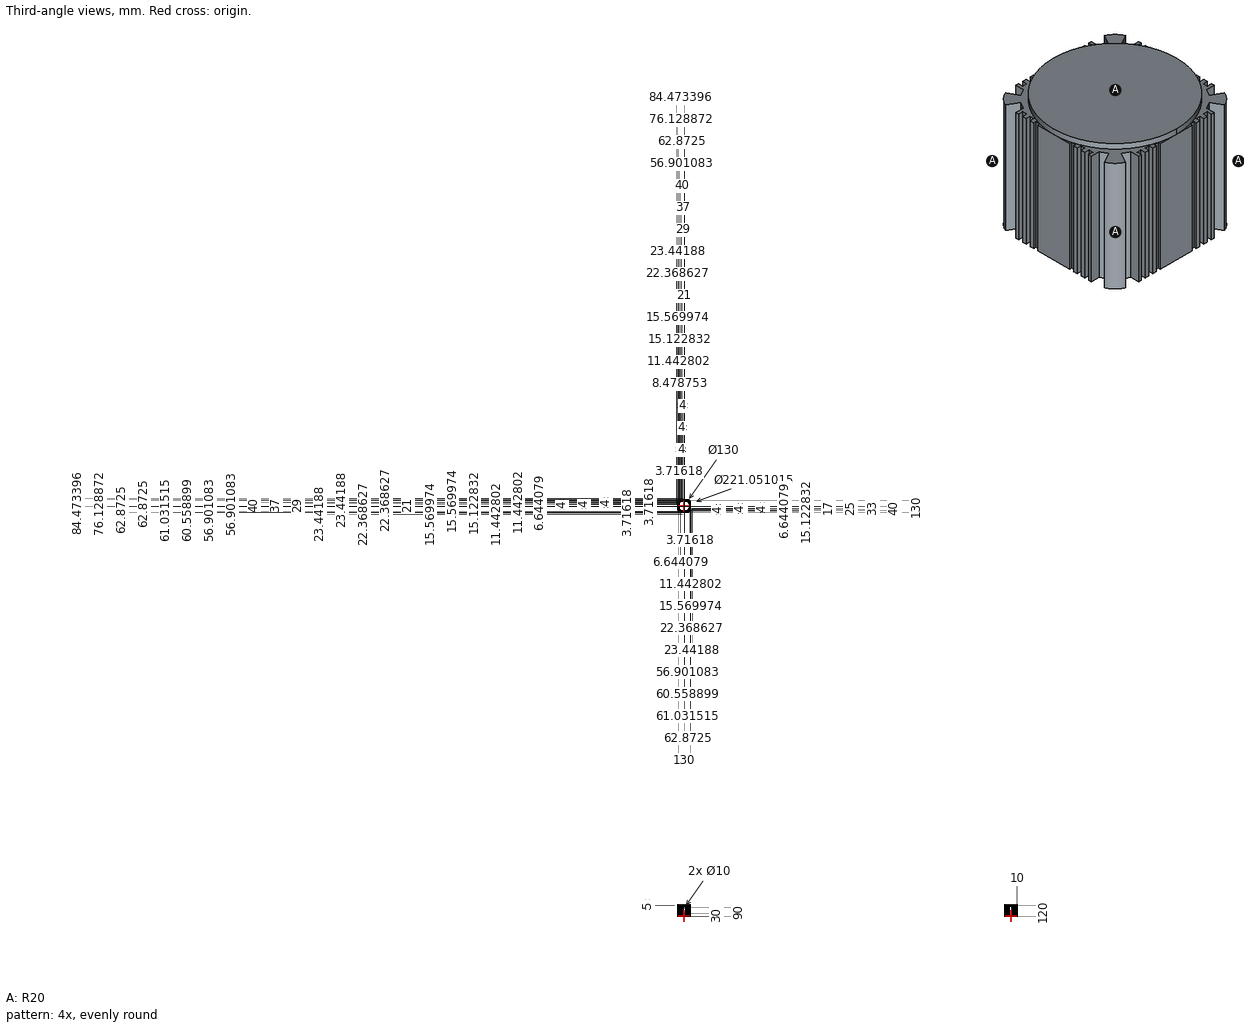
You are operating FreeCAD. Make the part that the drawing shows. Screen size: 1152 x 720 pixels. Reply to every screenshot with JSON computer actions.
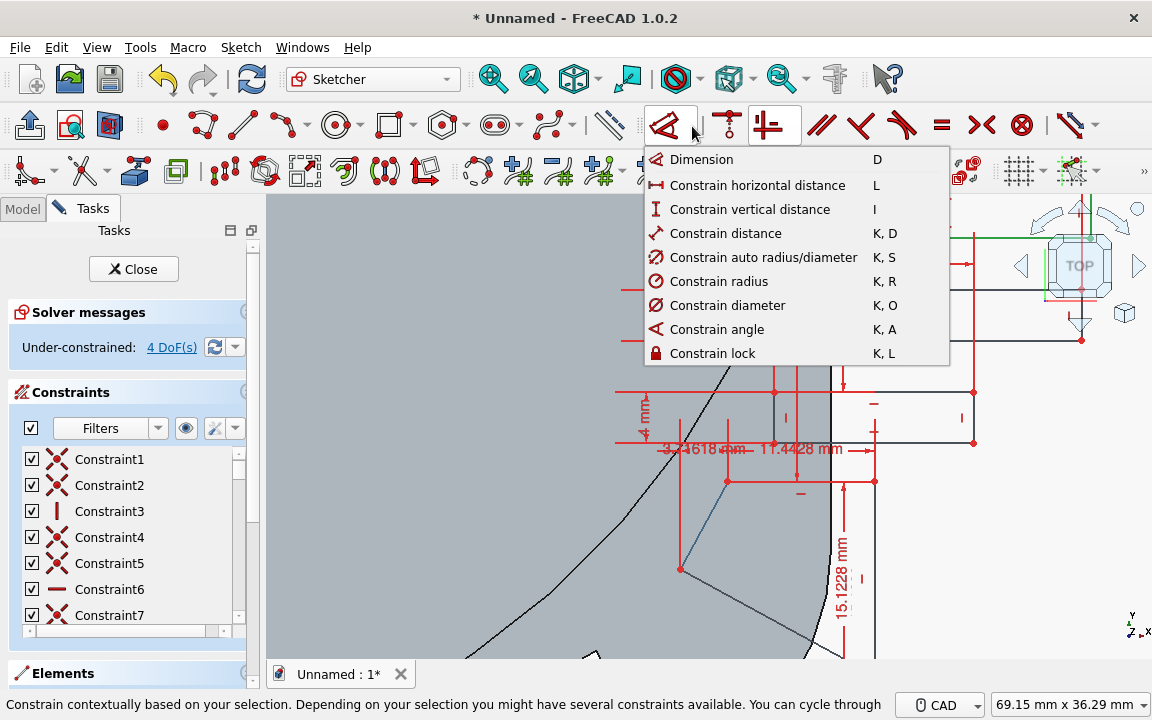
{"action": "left_click", "coordinate": [797, 209]}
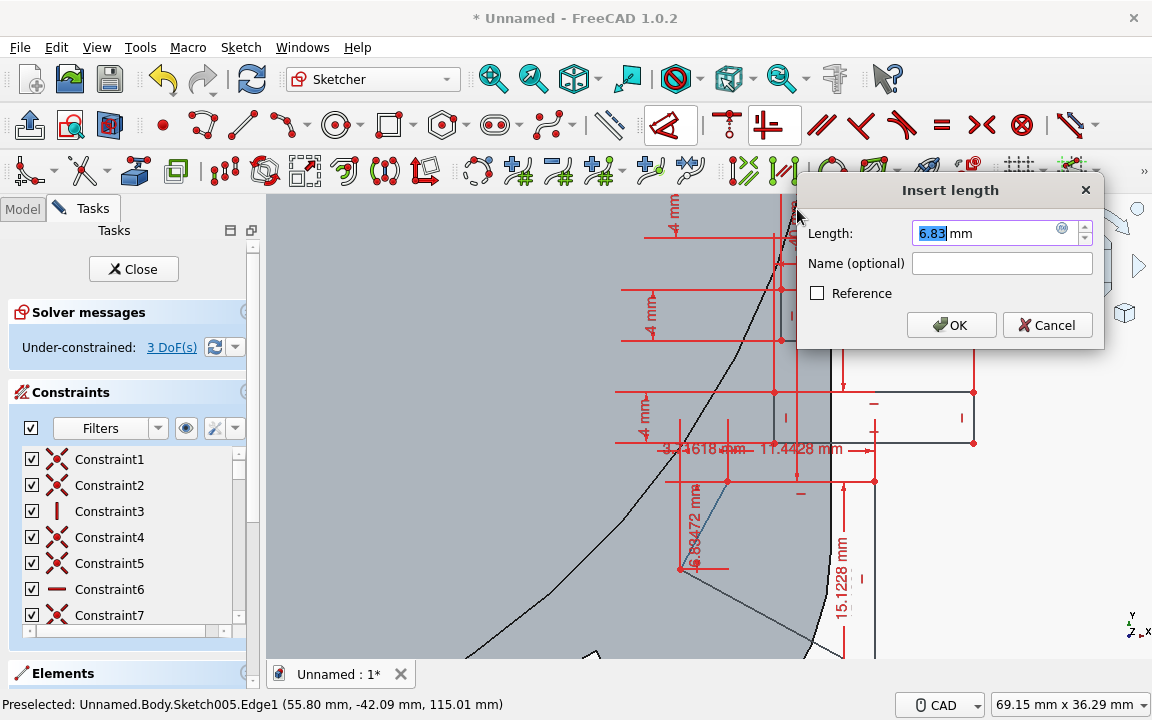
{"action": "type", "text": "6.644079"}
{"action": "key", "text": "Return"}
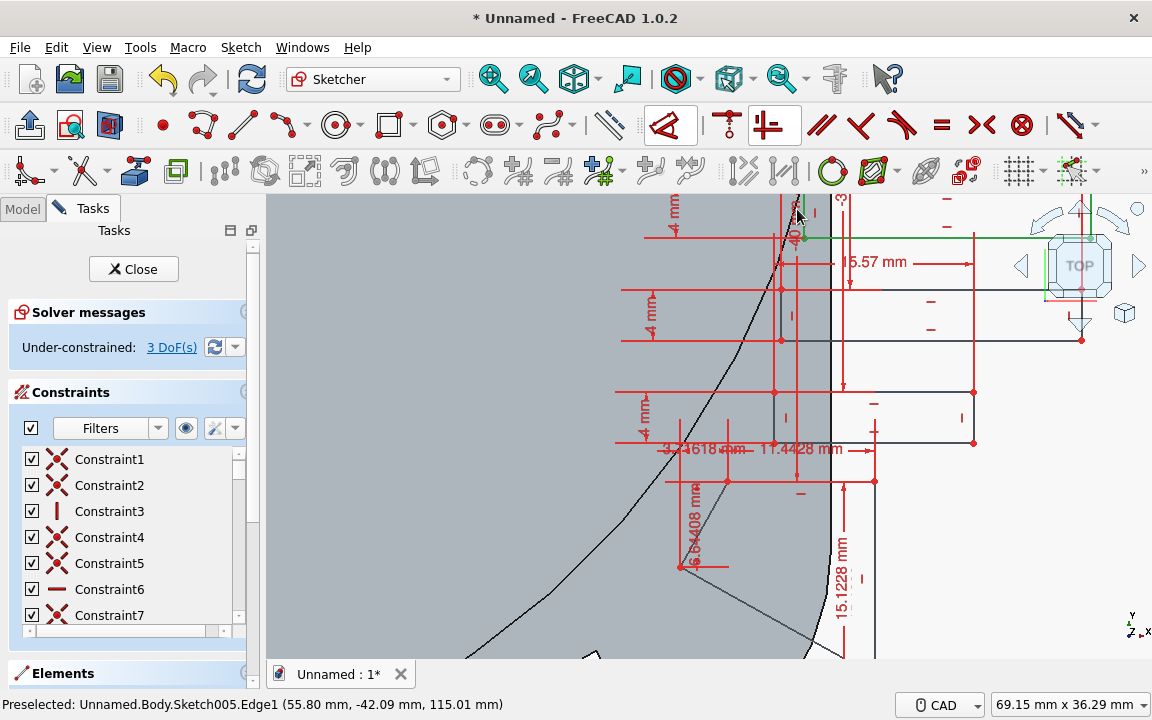
{"action": "left_click", "coordinate": [728, 482]}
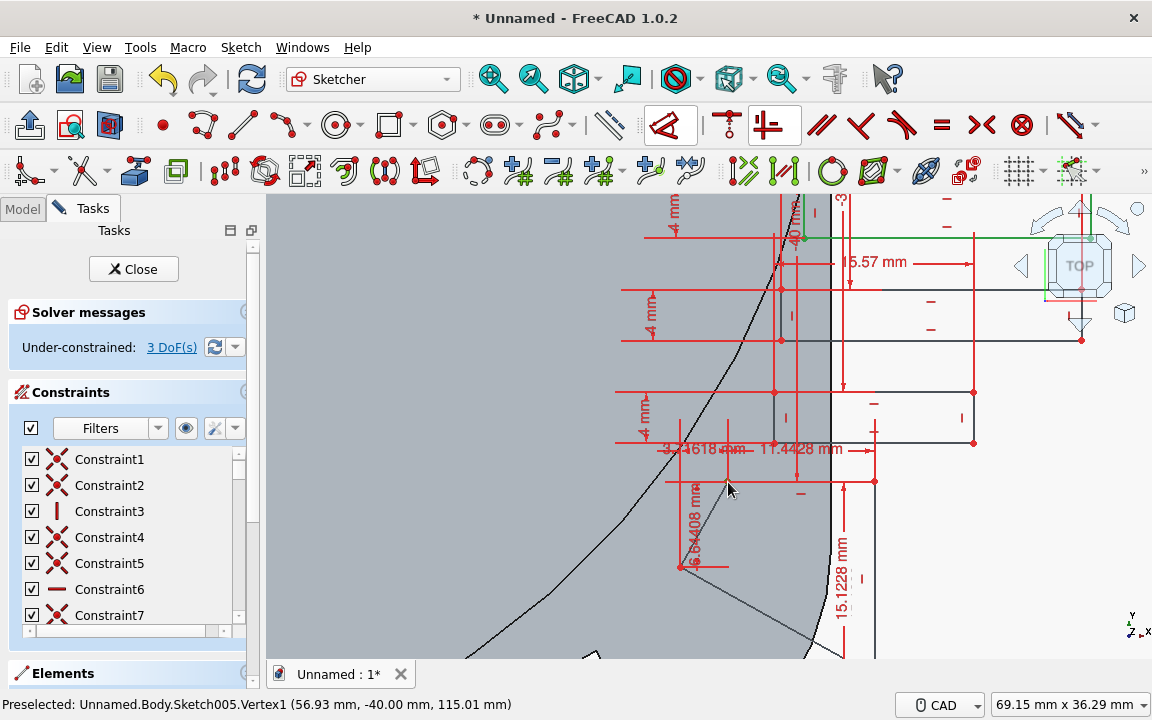
{"action": "left_click", "coordinate": [692, 126]}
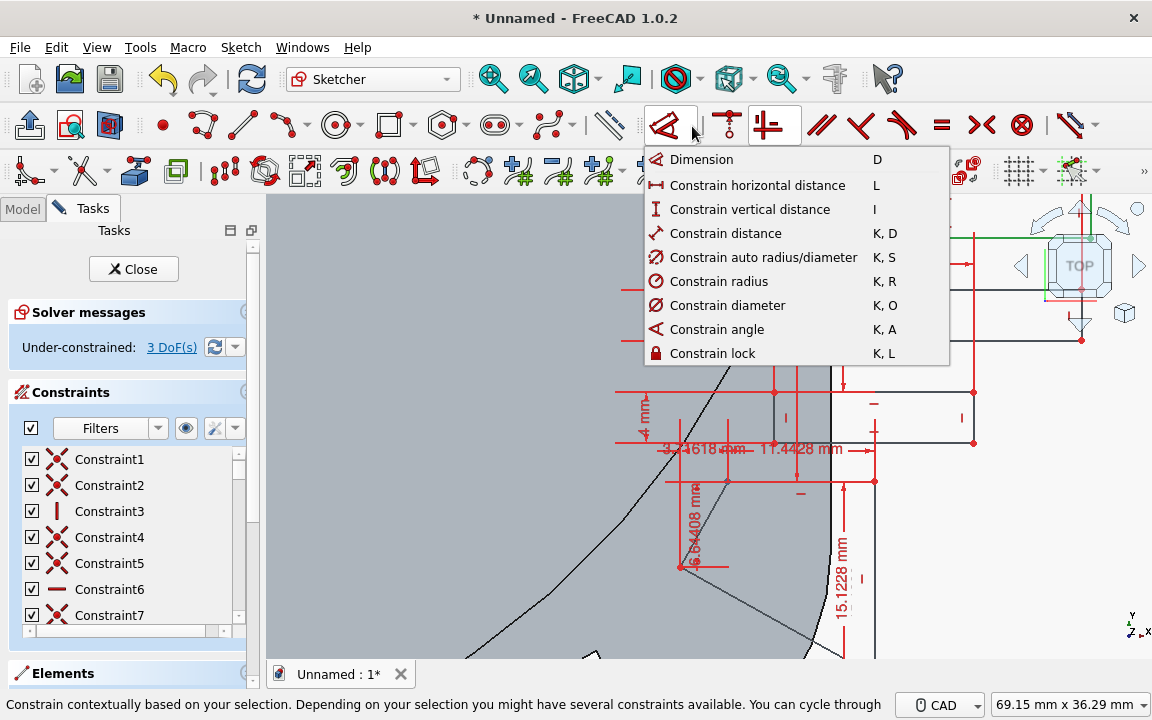
{"action": "left_click", "coordinate": [797, 185]}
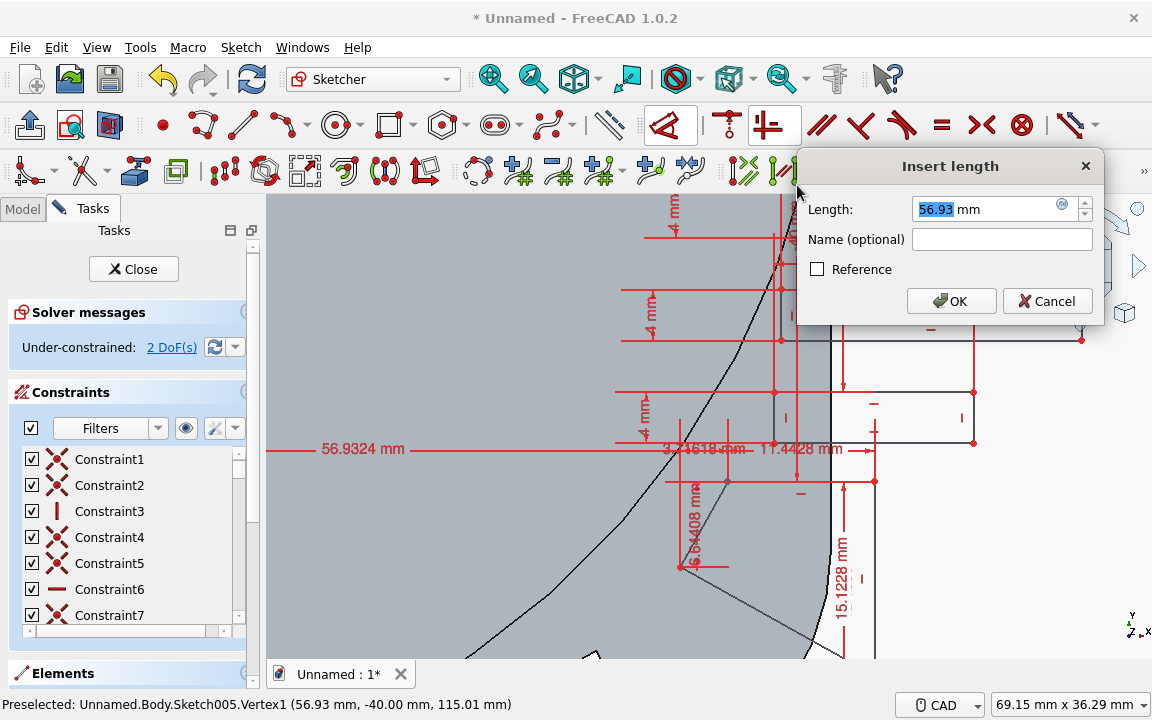
{"action": "type", "text": "56.901083"}
{"action": "key", "text": "Return"}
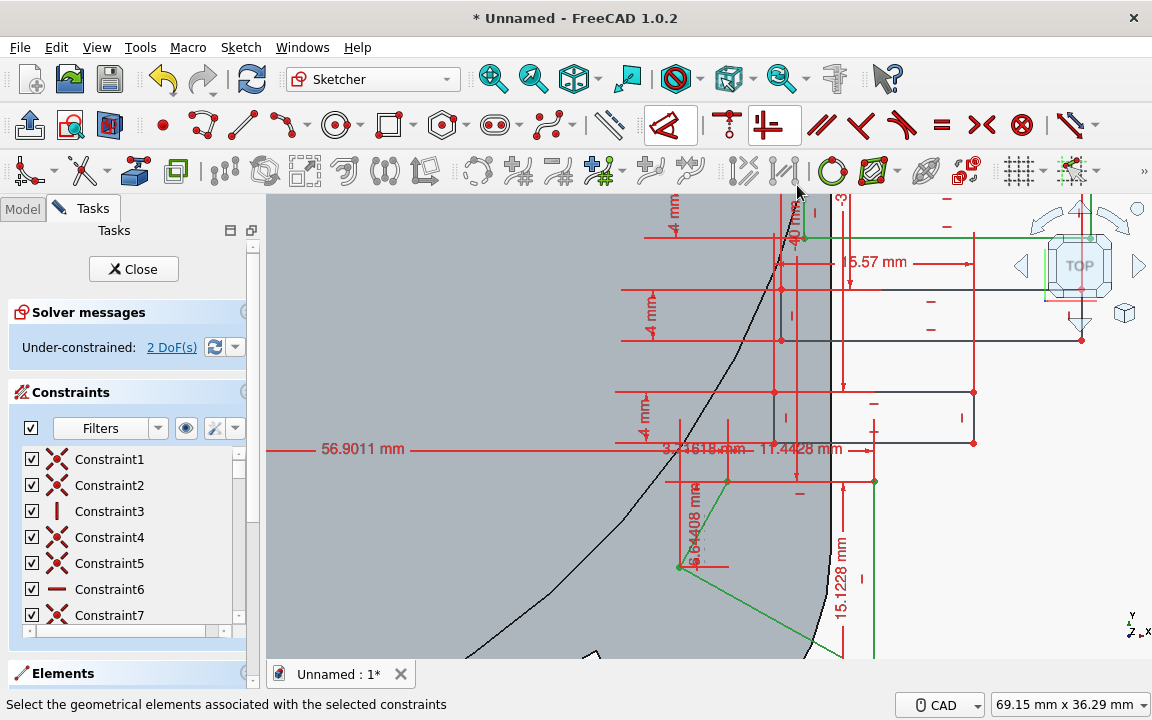
{"action": "left_click", "coordinate": [774, 392]}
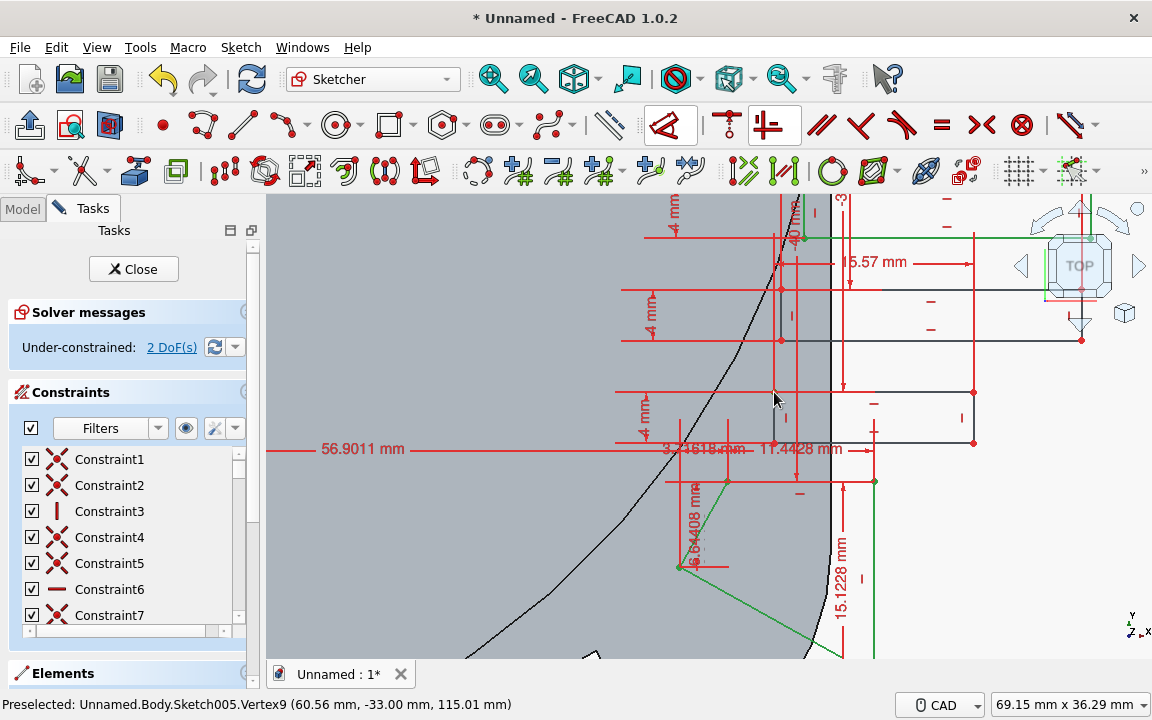
{"action": "key", "text": "l"}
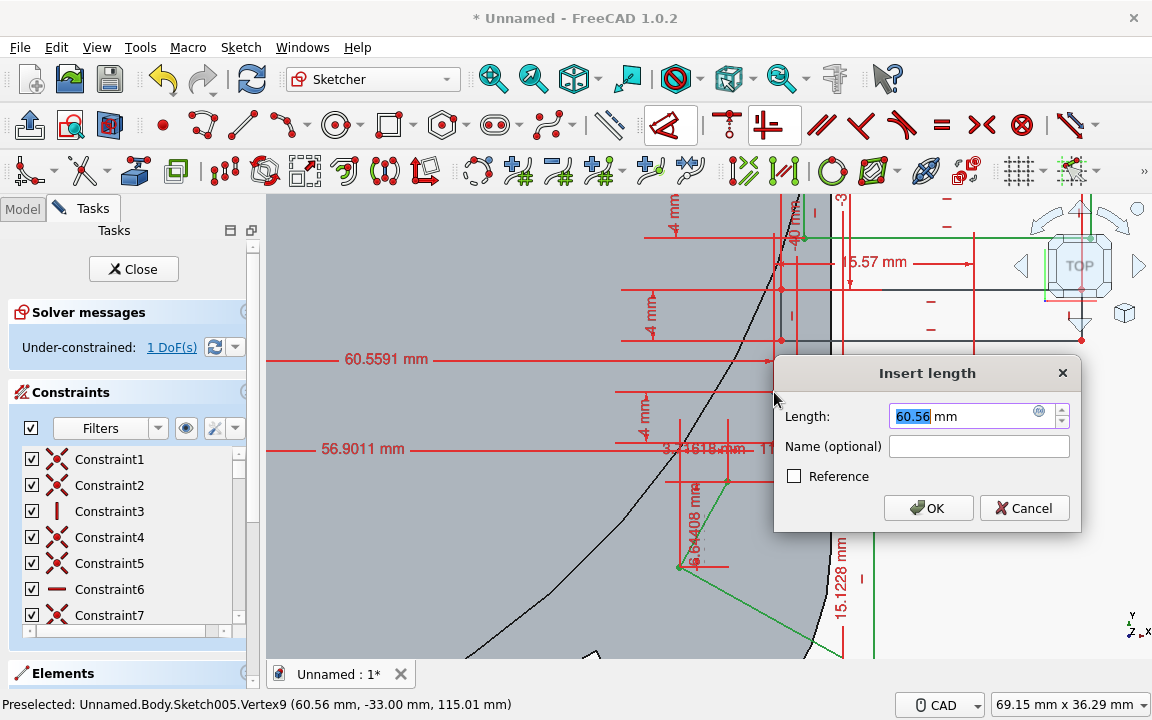
{"action": "type", "text": "60.558899"}
{"action": "key", "text": "Return"}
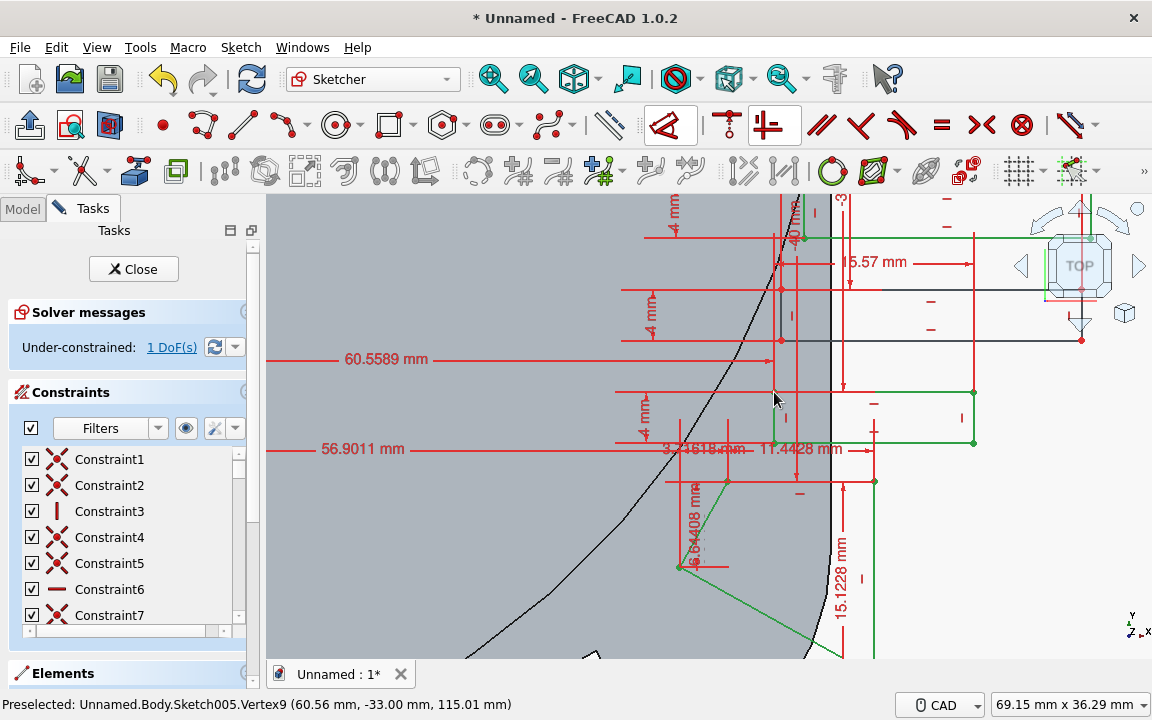
{"action": "left_click", "coordinate": [781, 290]}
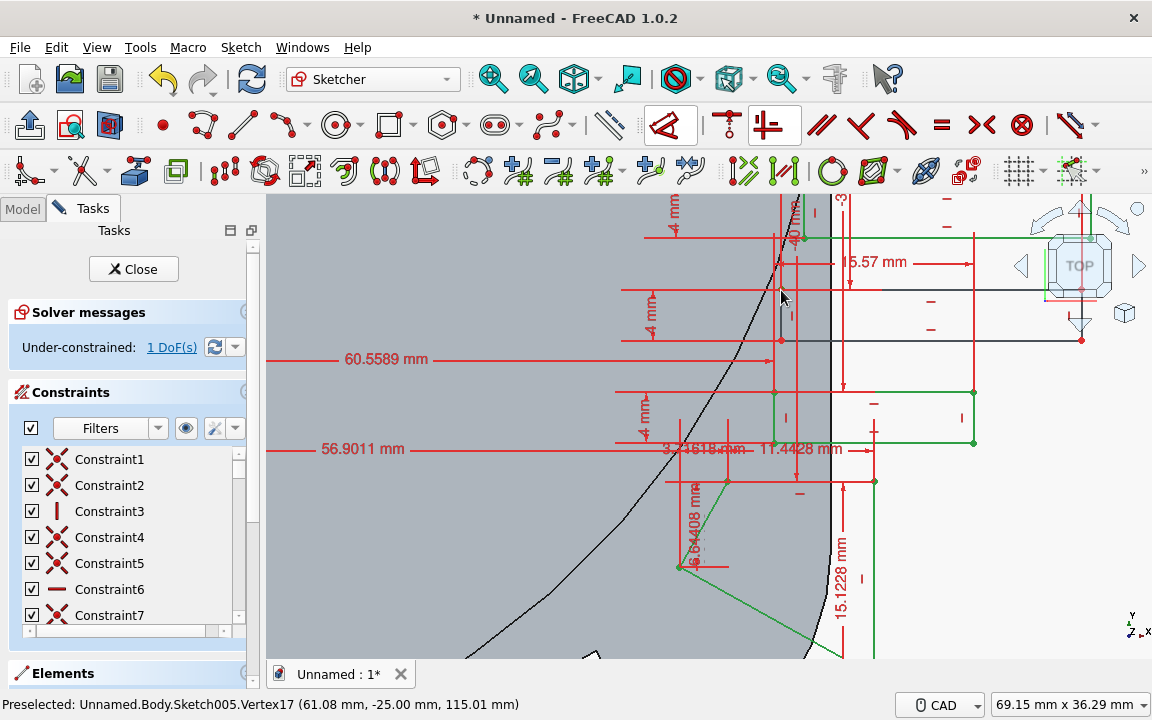
{"action": "key", "text": "l"}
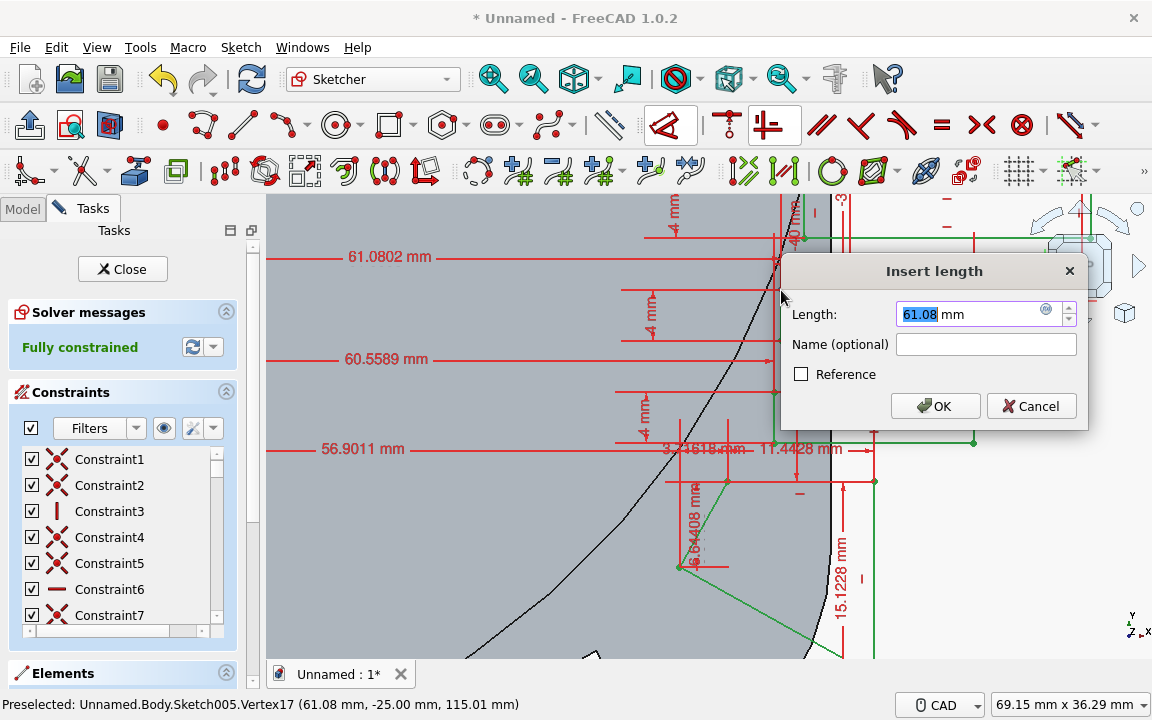
{"action": "type", "text": "61.031515"}
{"action": "key", "text": "Return"}